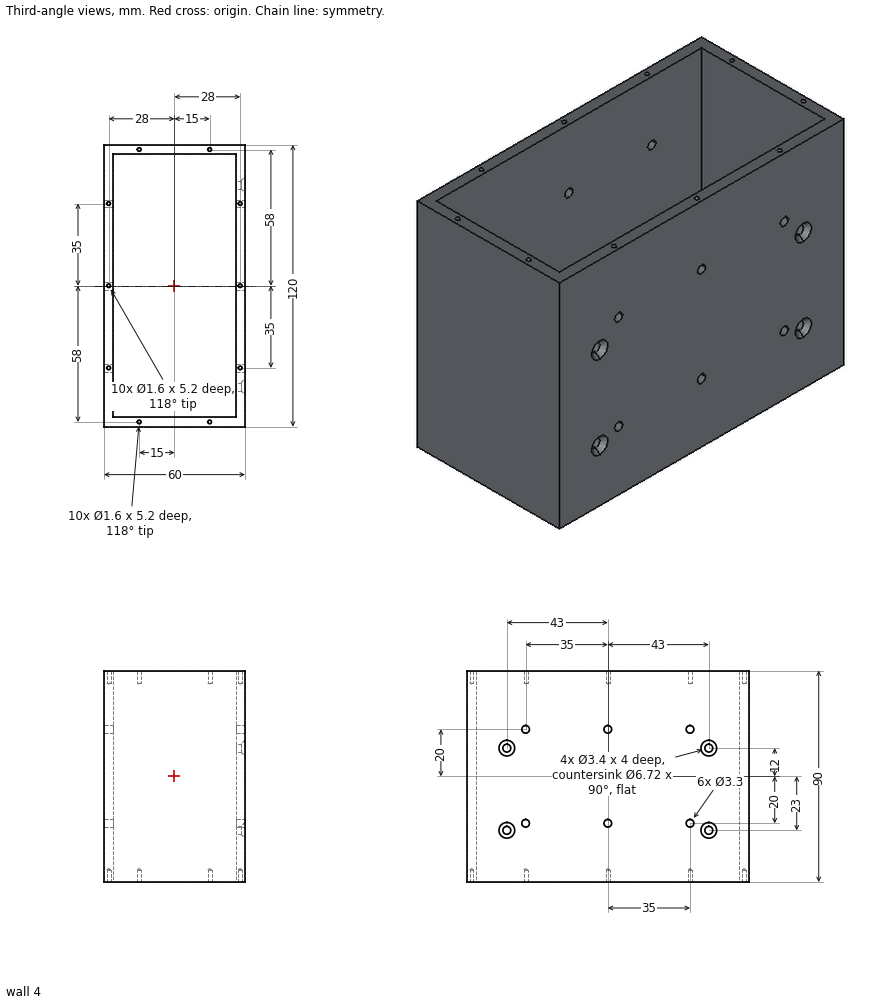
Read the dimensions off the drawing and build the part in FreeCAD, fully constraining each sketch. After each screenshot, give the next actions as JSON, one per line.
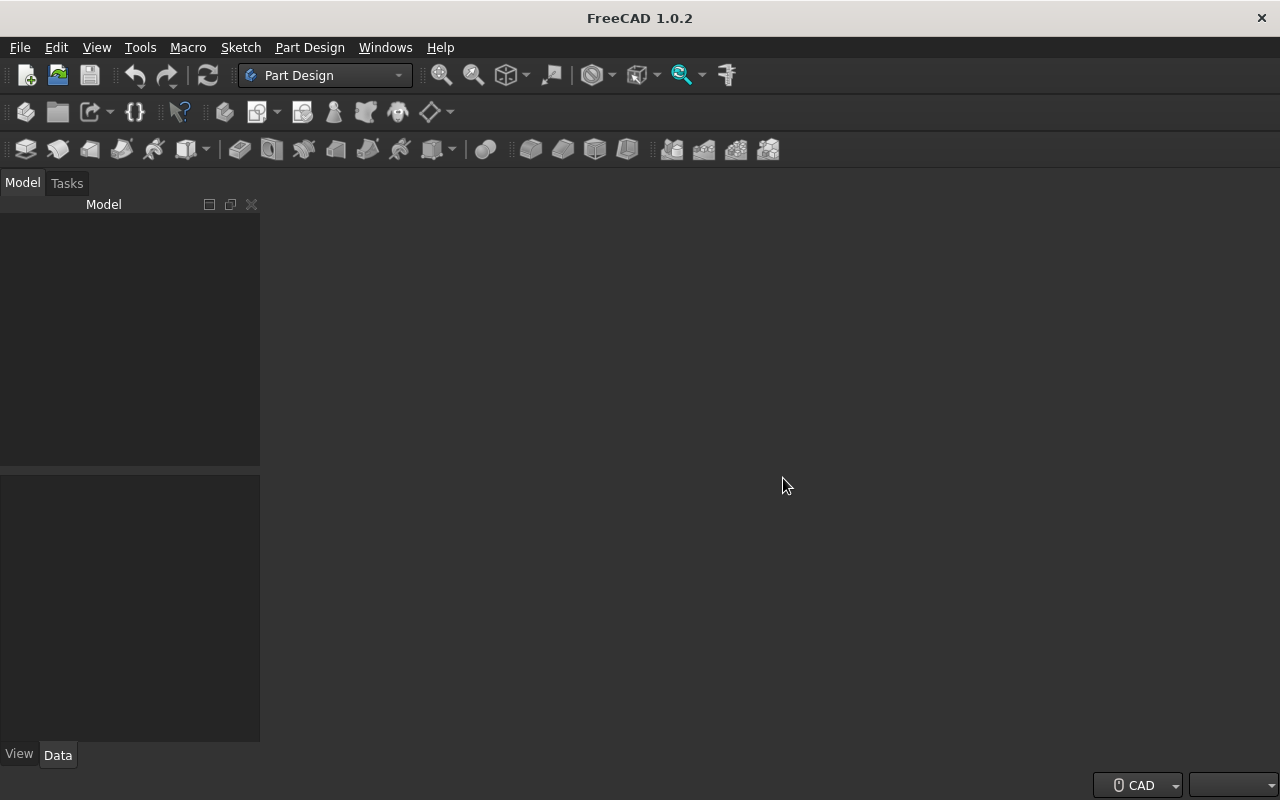
{"action": "left_click", "coordinate": [26, 76]}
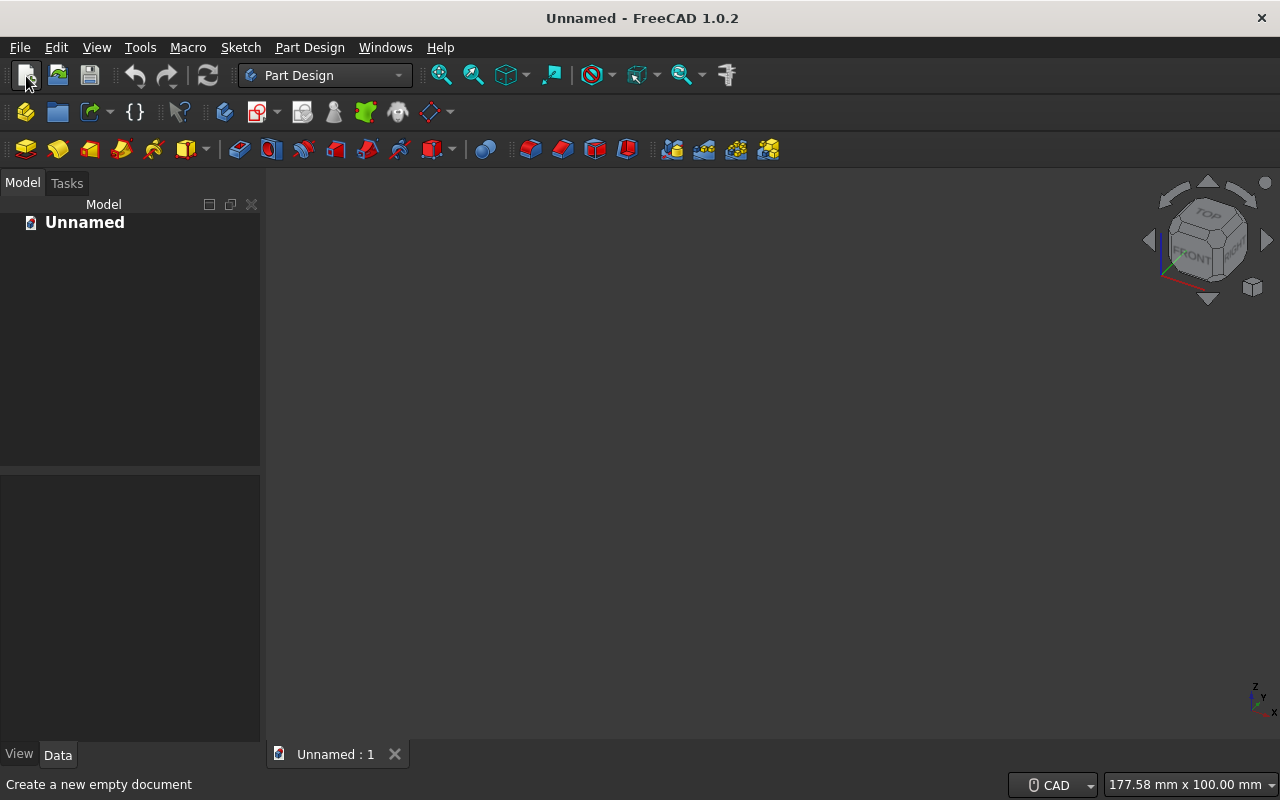
{"action": "left_click", "coordinate": [258, 112]}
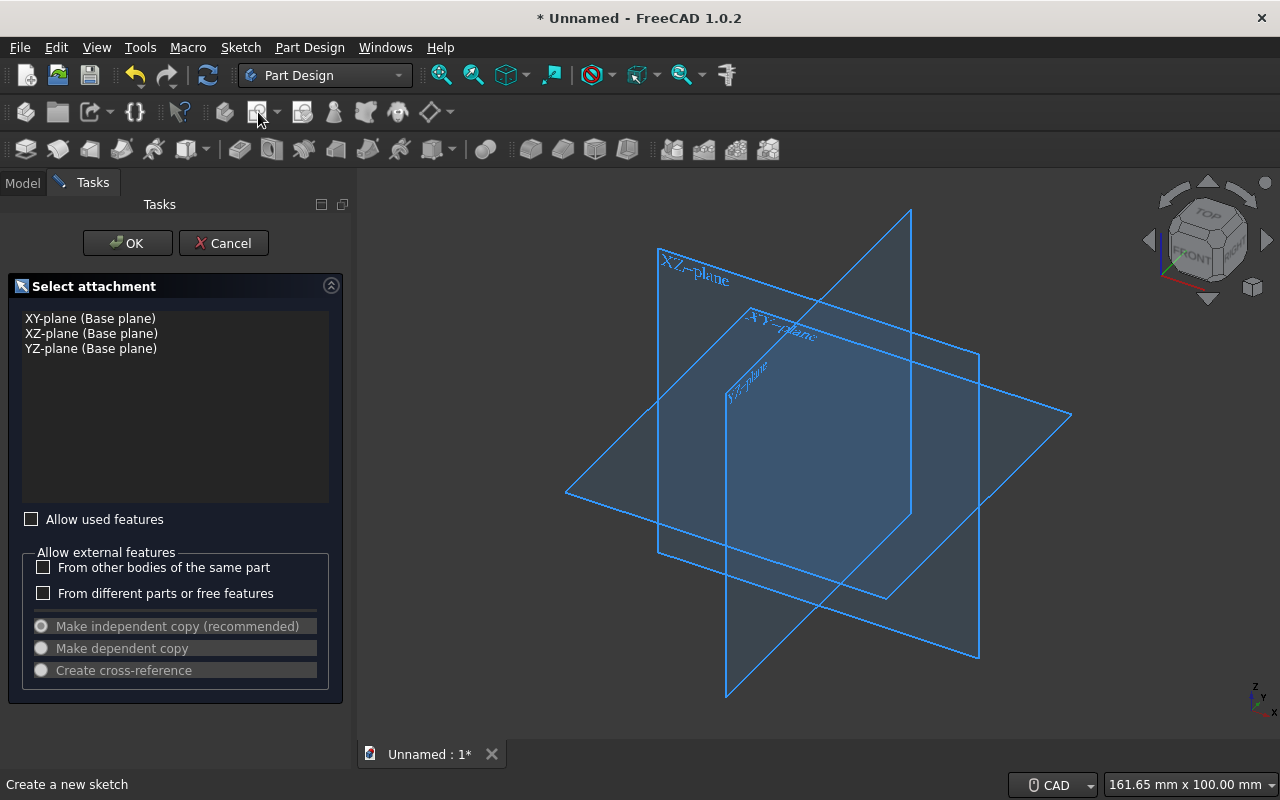
{"action": "left_click", "coordinate": [82, 318]}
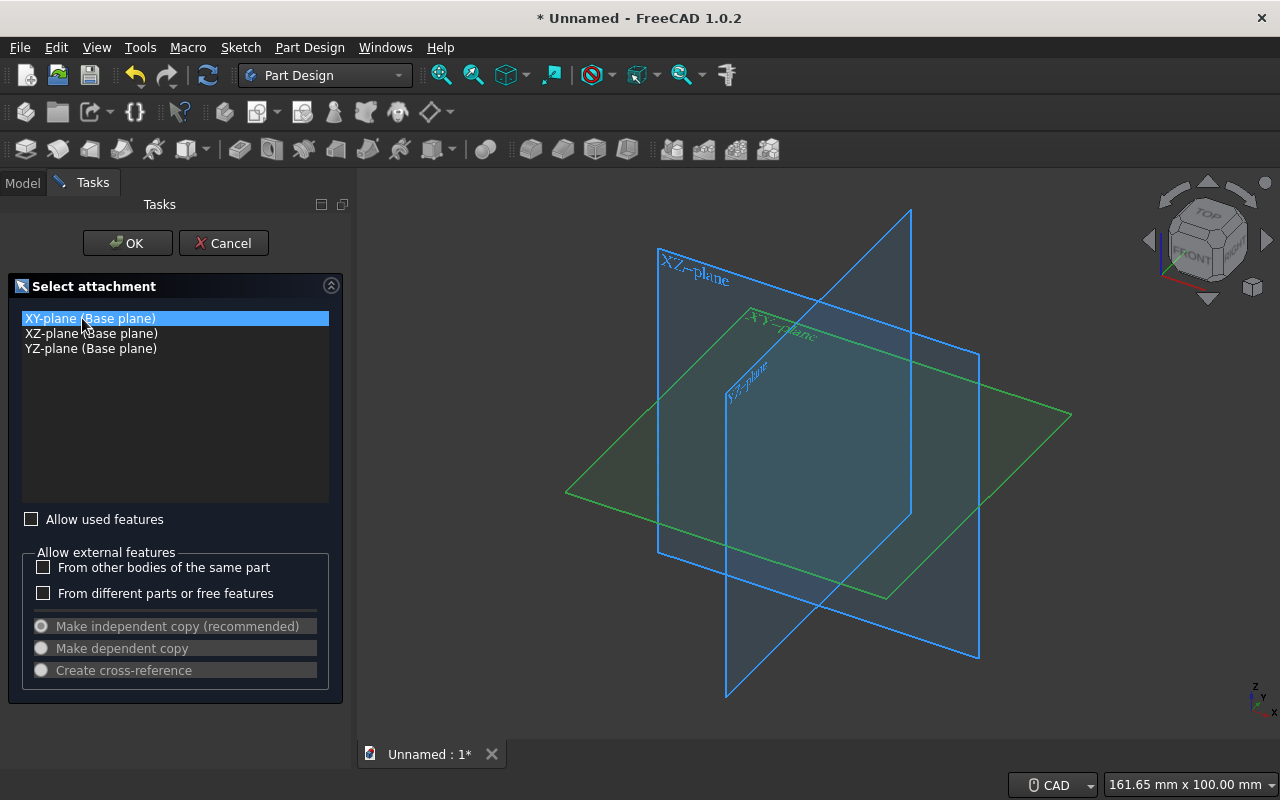
{"action": "left_click", "coordinate": [128, 243]}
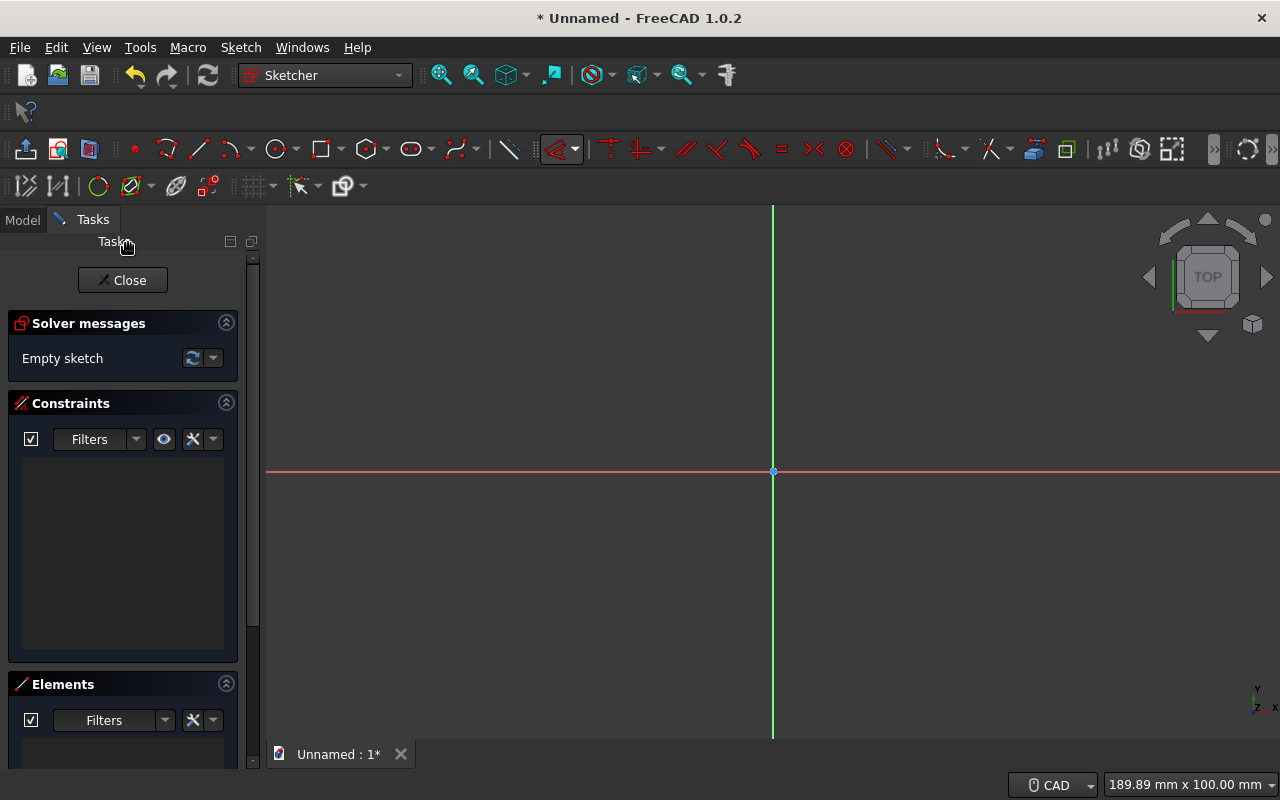
{"action": "scroll", "coordinate": [621, 472], "scroll_direction": "down", "scroll_amount": 3}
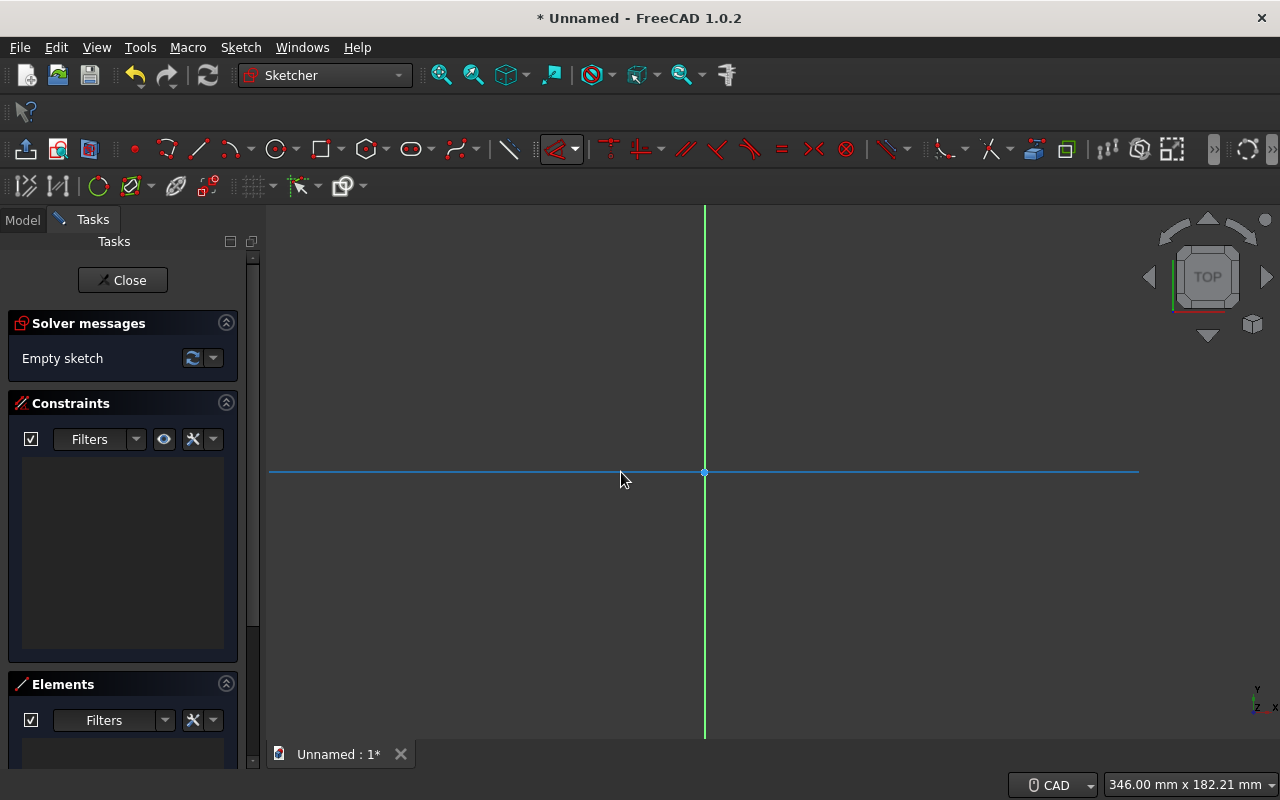
{"action": "left_click", "coordinate": [344, 150]}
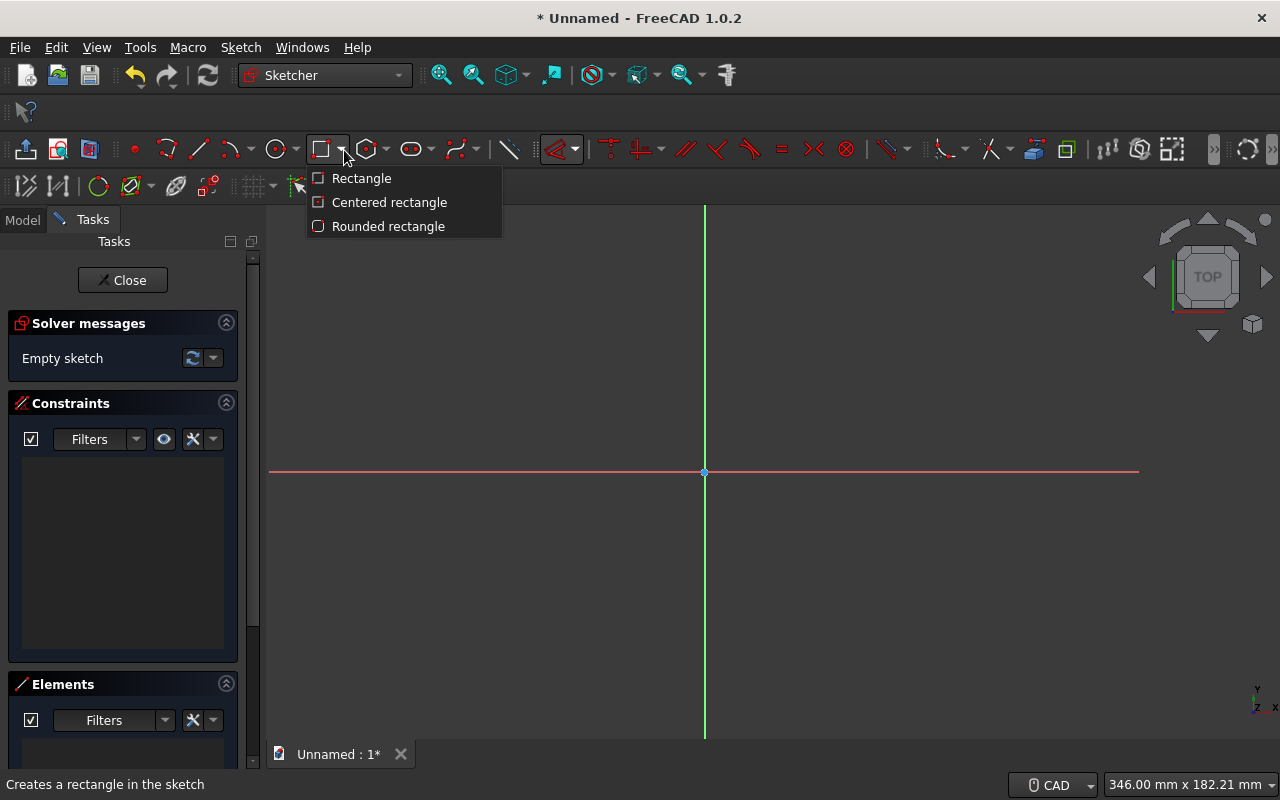
{"action": "left_click", "coordinate": [404, 202]}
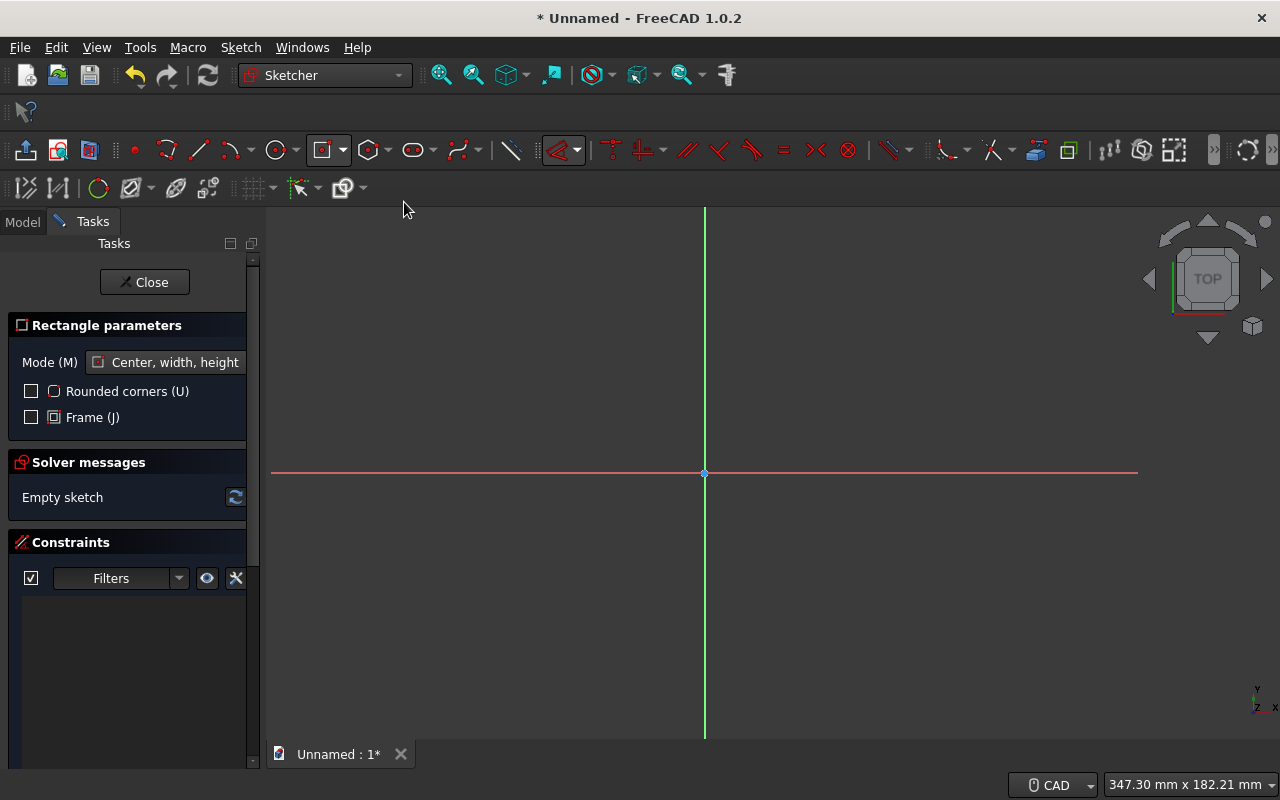
{"action": "left_click", "coordinate": [705, 473]}
{"action": "mouse_move", "coordinate": [792, 298]}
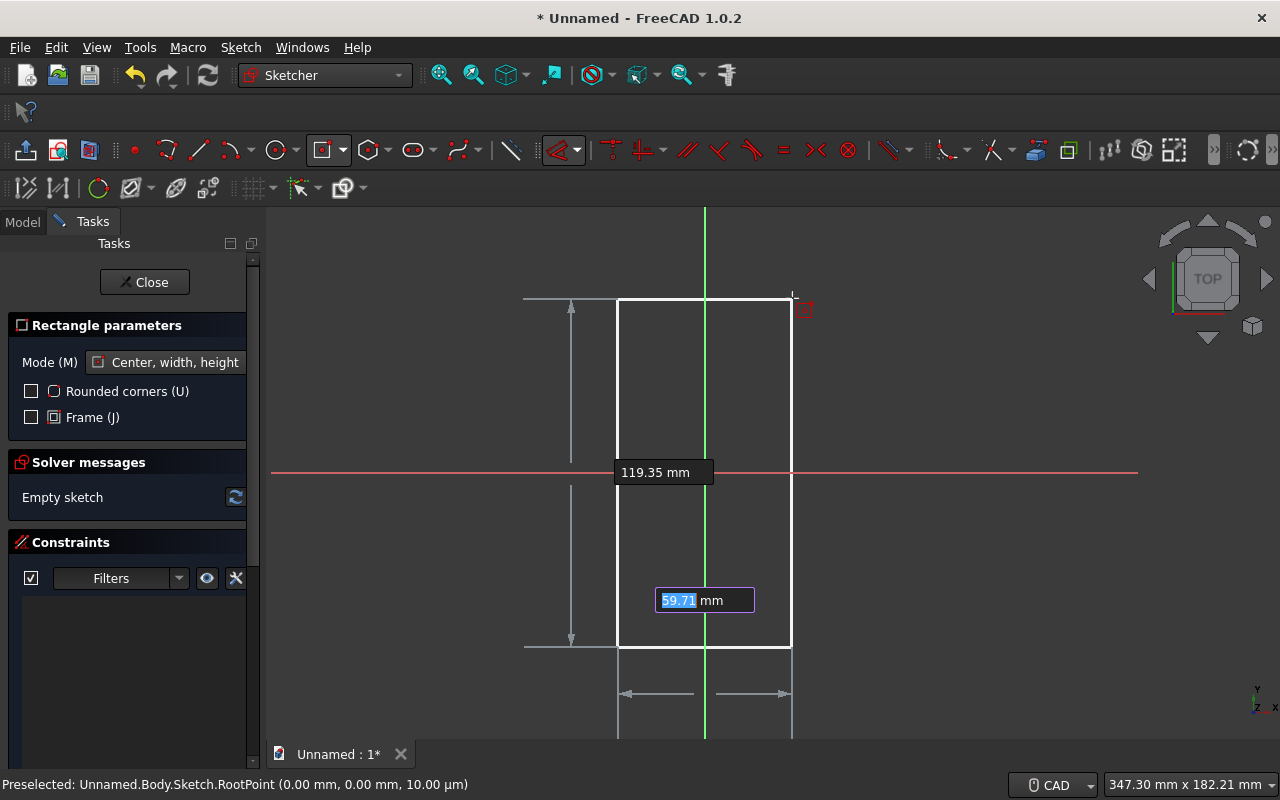
{"action": "type", "text": "60"}
{"action": "key", "text": "Tab"}
{"action": "type", "text": "120"}
{"action": "key", "text": "Return"}
{"action": "key", "text": "Escape"}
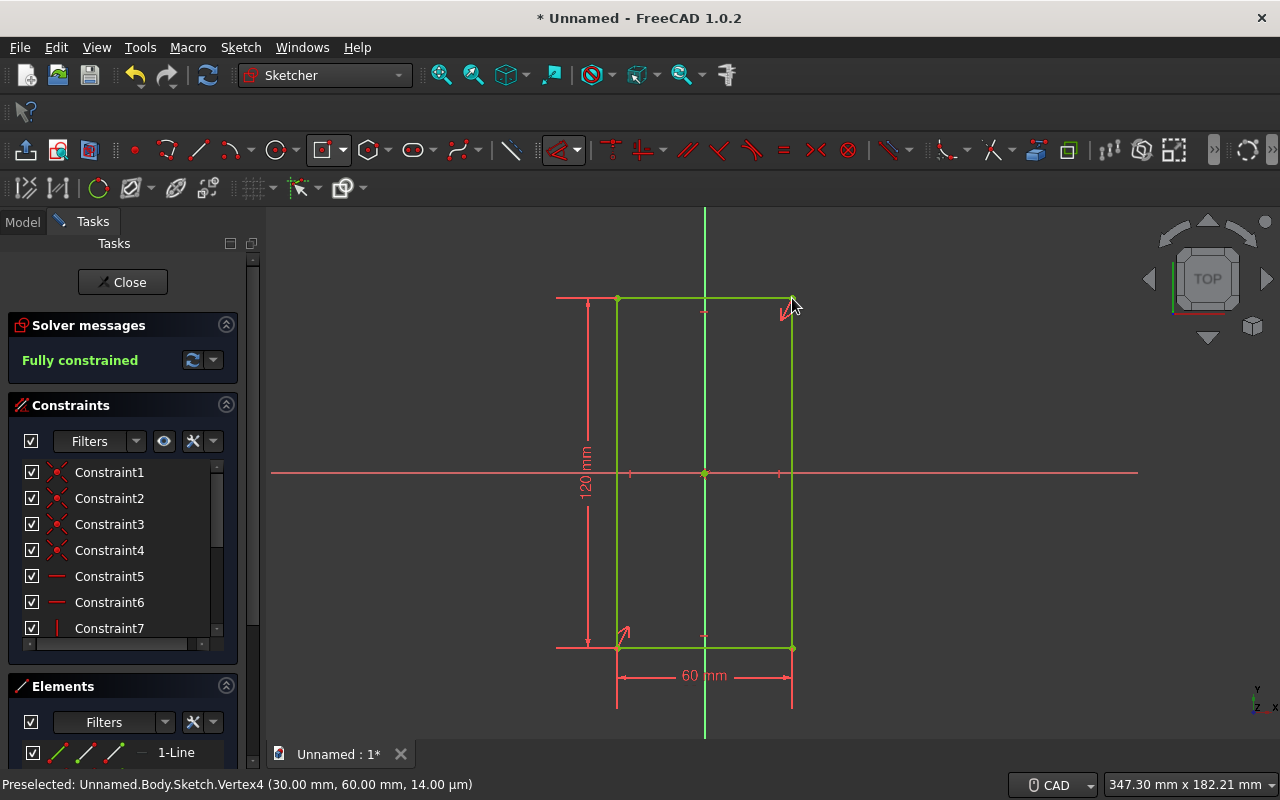
{"action": "left_click", "coordinate": [123, 282]}